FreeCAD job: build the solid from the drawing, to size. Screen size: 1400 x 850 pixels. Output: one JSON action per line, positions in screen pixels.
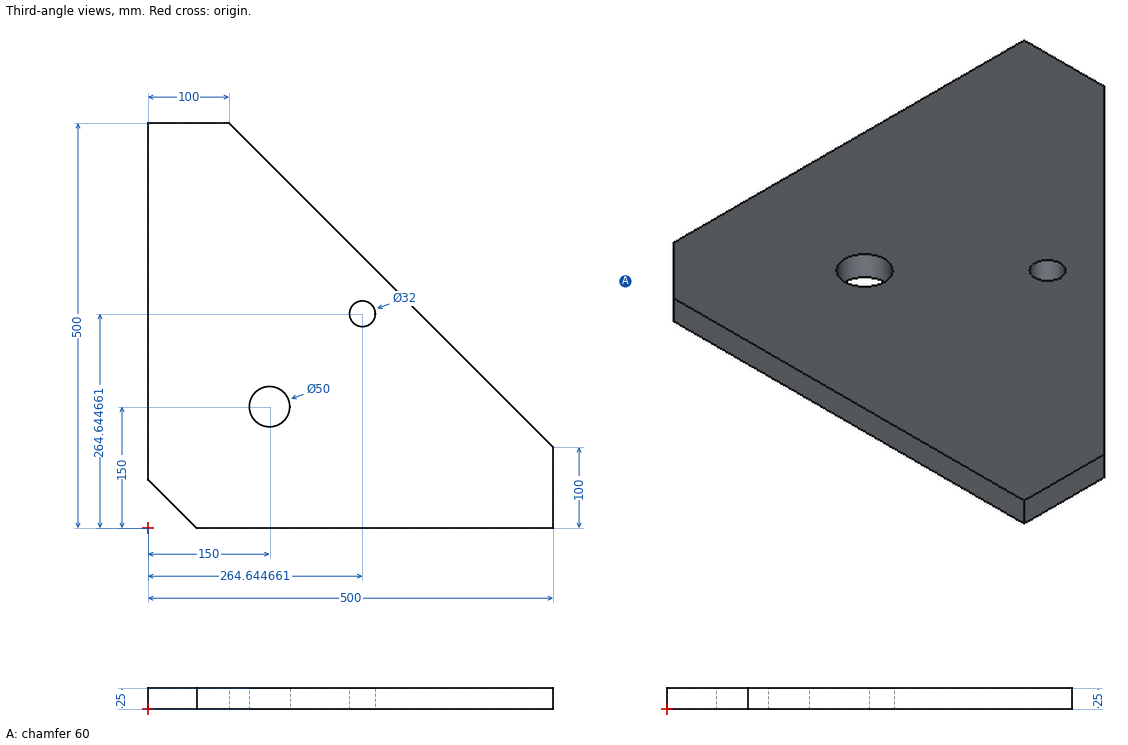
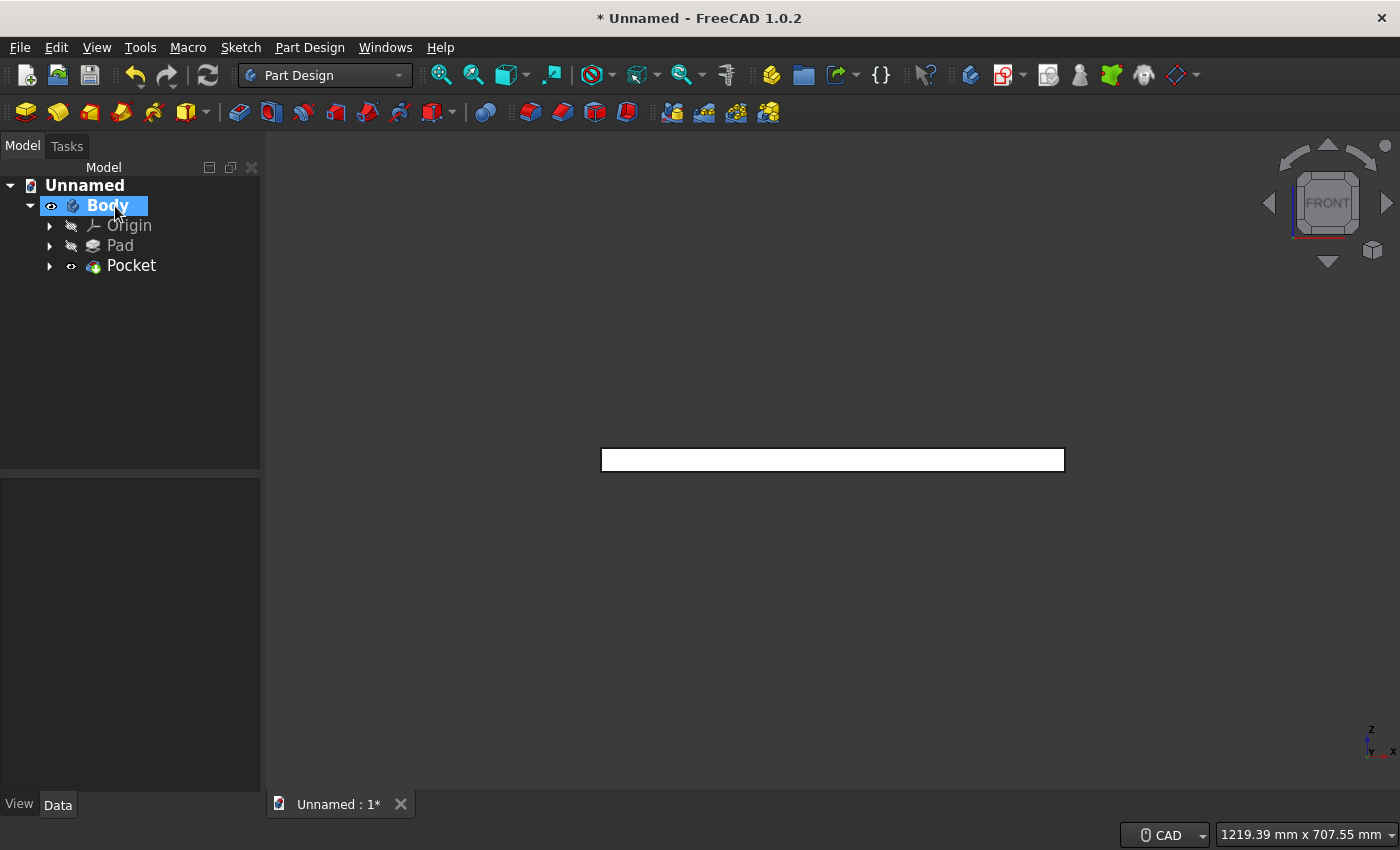
{"action": "left_click", "coordinate": [442, 76]}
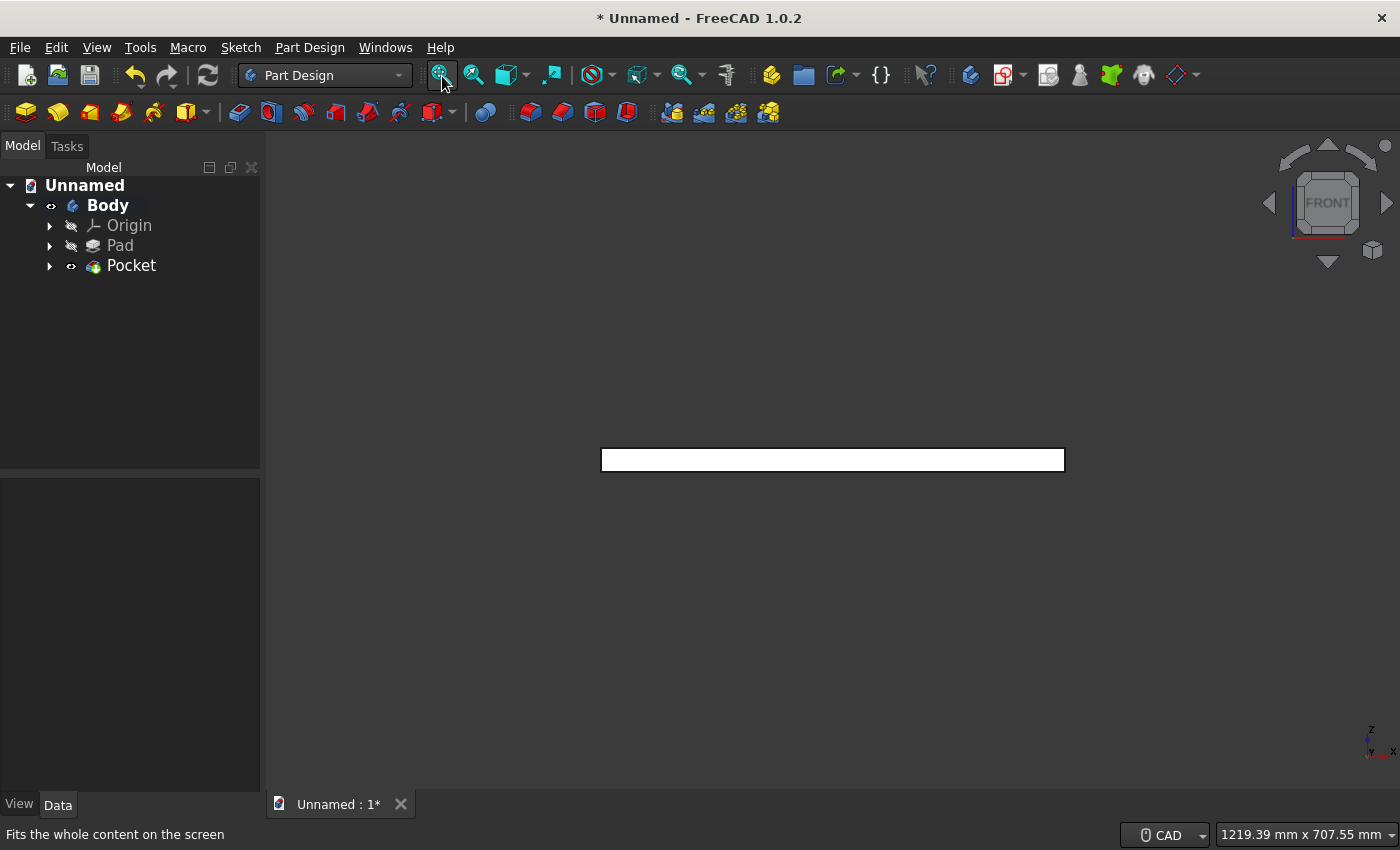
{"action": "left_click", "coordinate": [601, 459]}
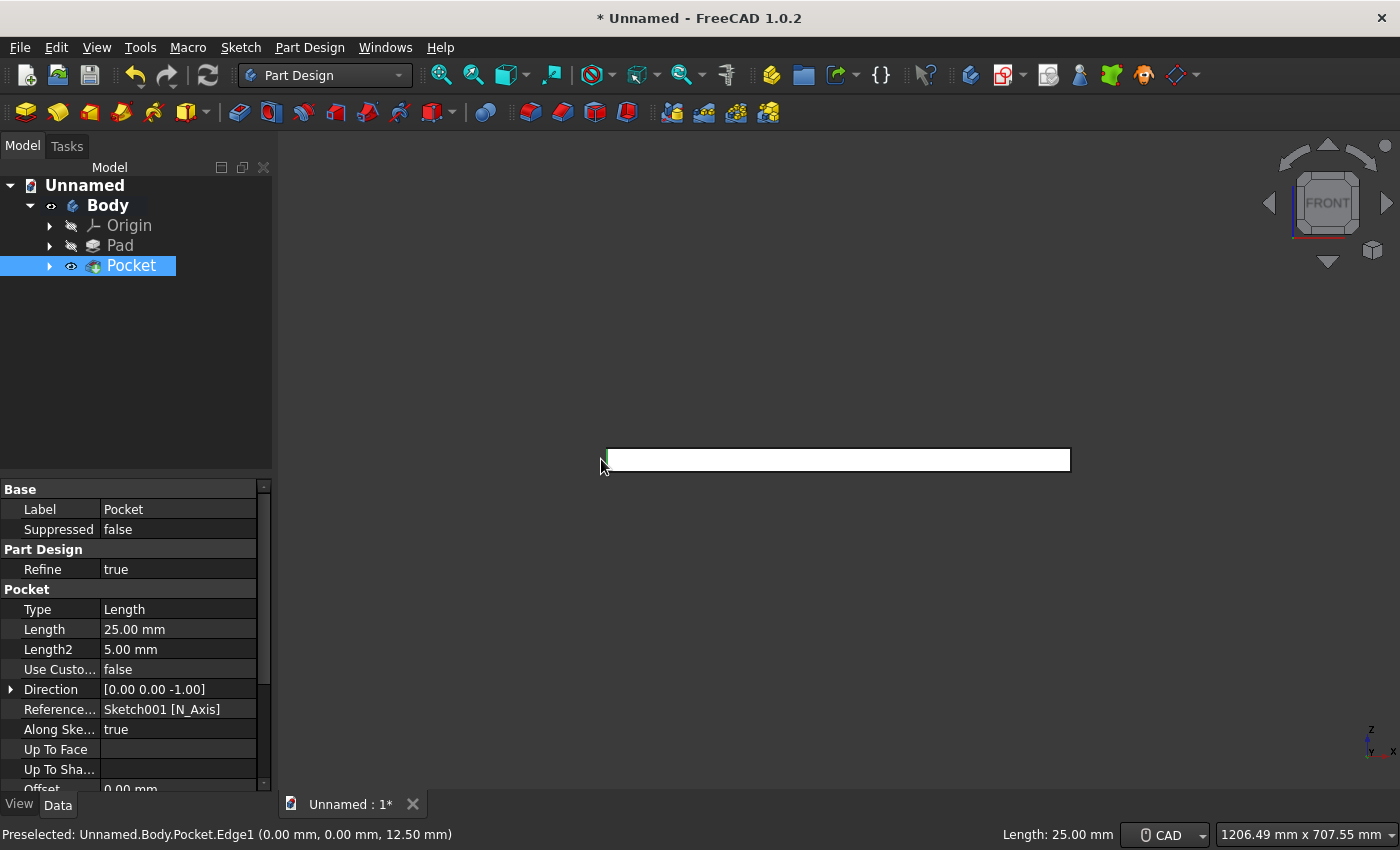
{"action": "left_click", "coordinate": [564, 112]}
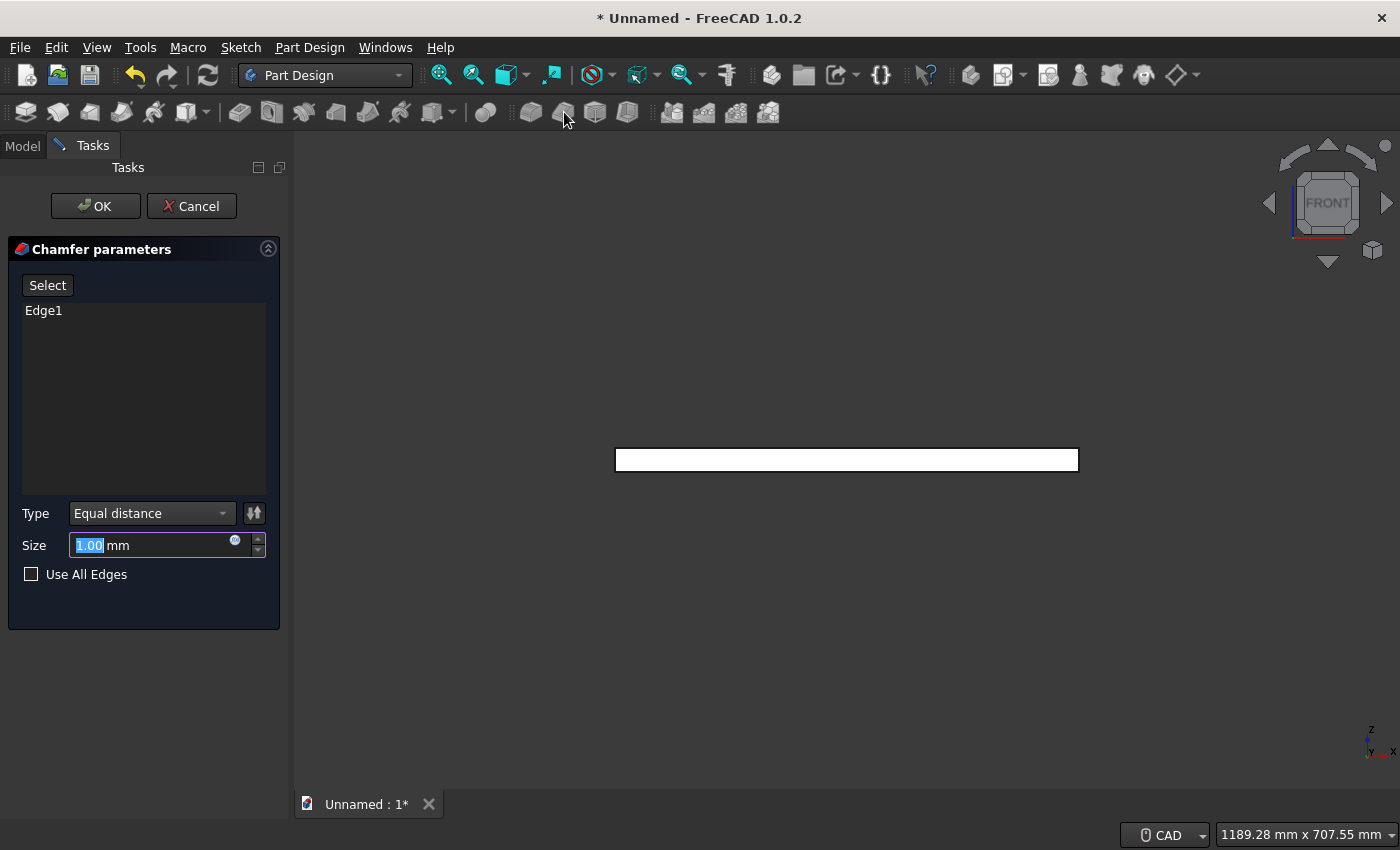
{"action": "type", "text": "60"}
{"action": "key", "text": "Tab"}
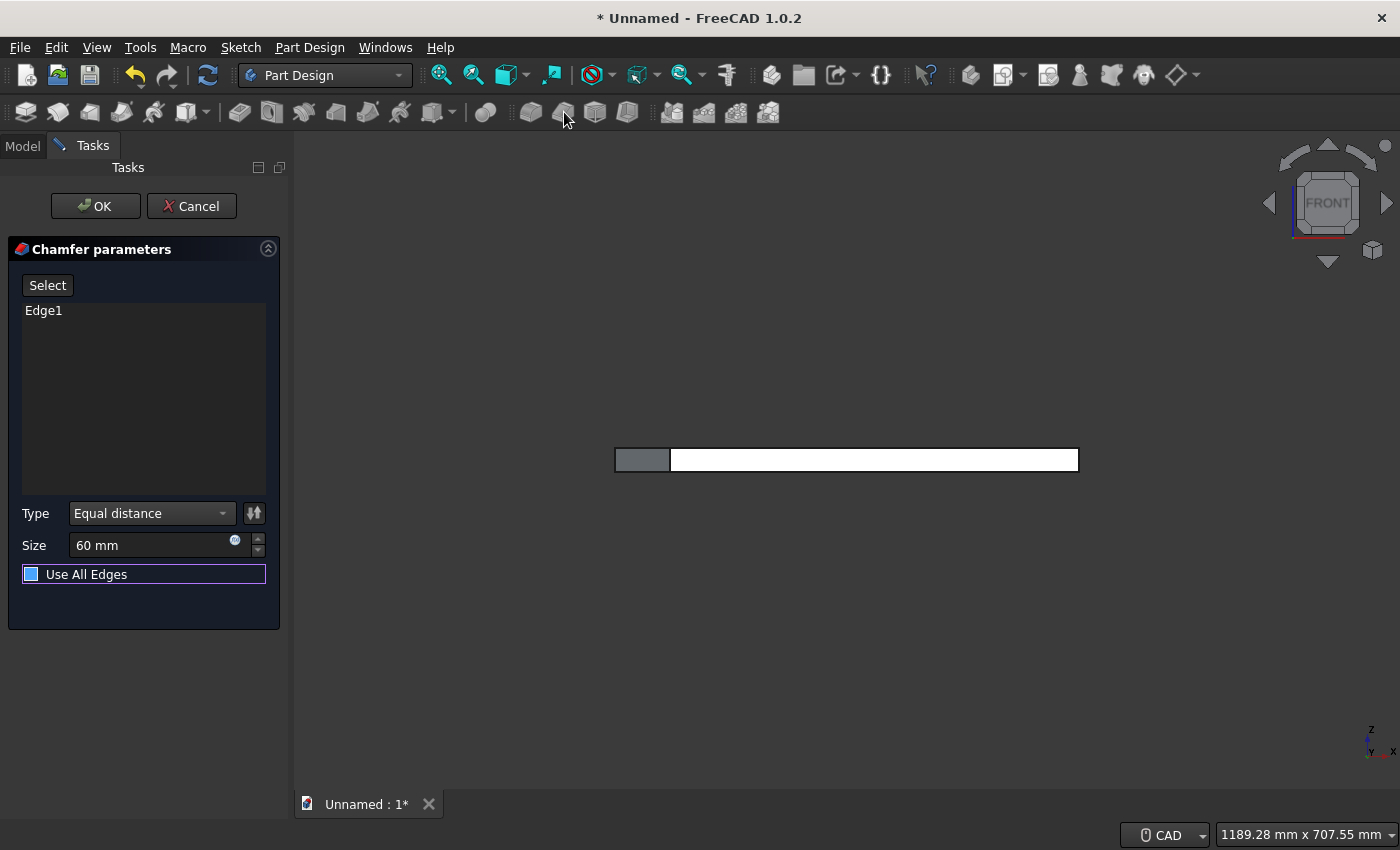
{"action": "left_click", "coordinate": [96, 206]}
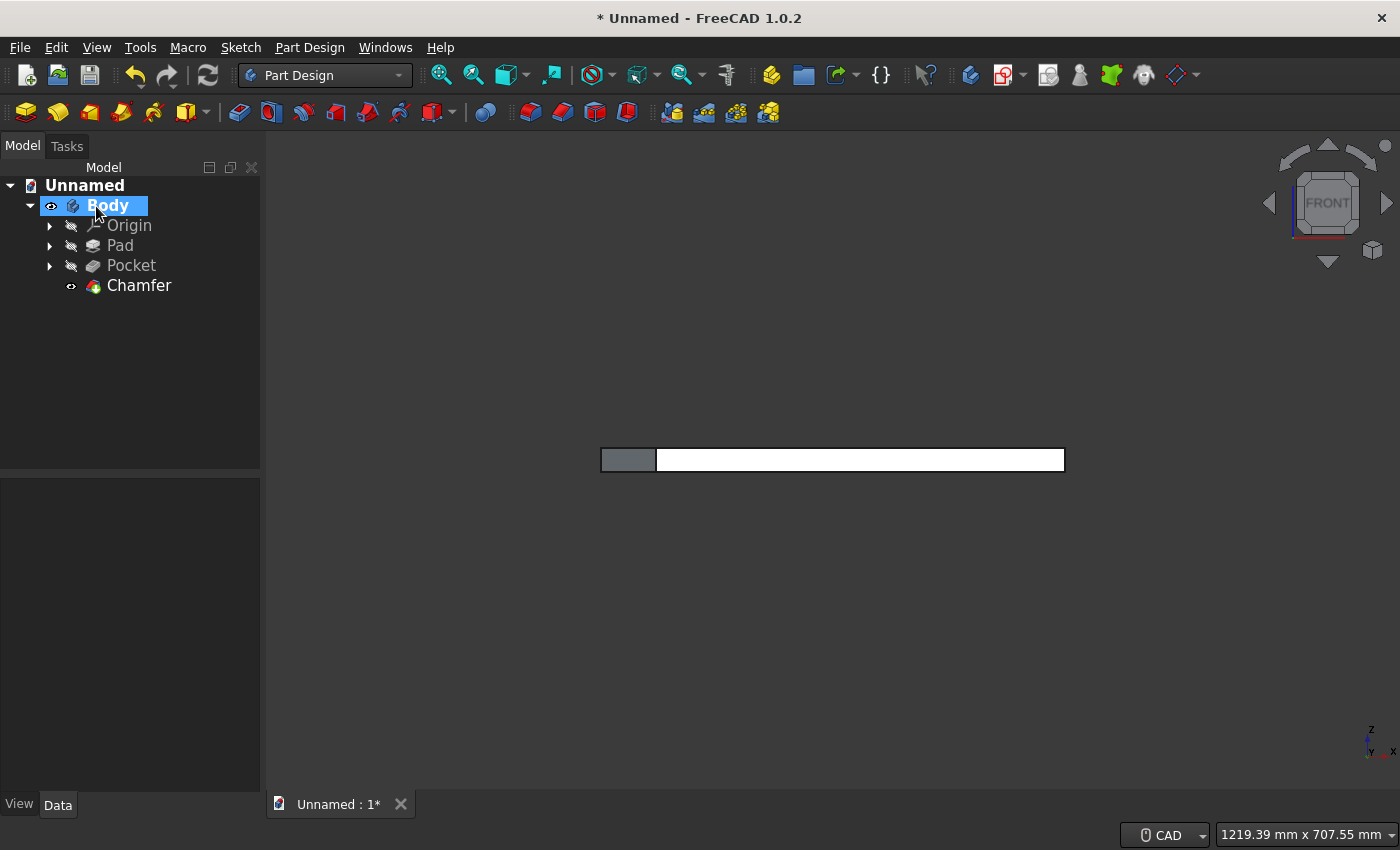
{"action": "left_click", "coordinate": [442, 76]}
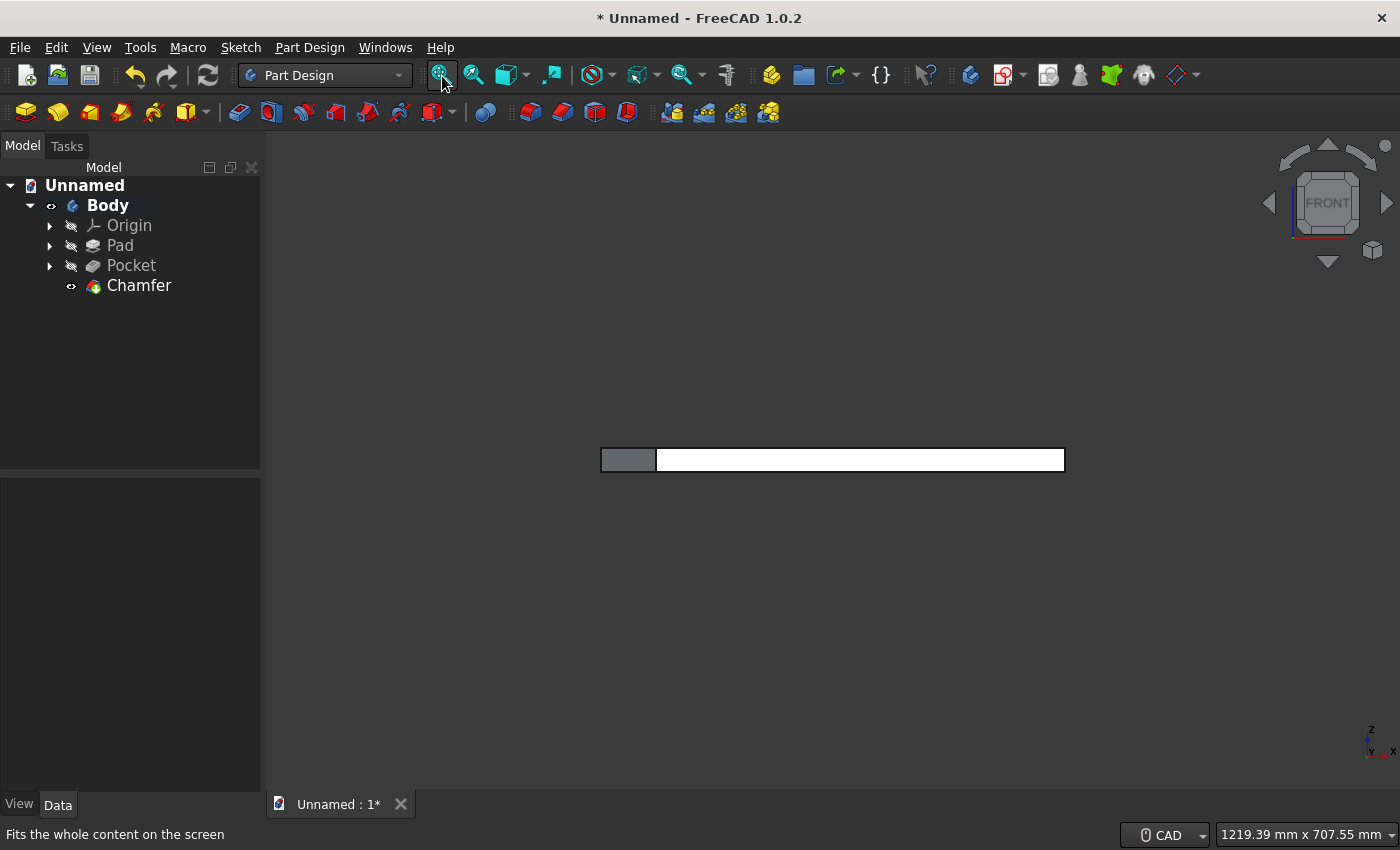
{"action": "key", "text": "0"}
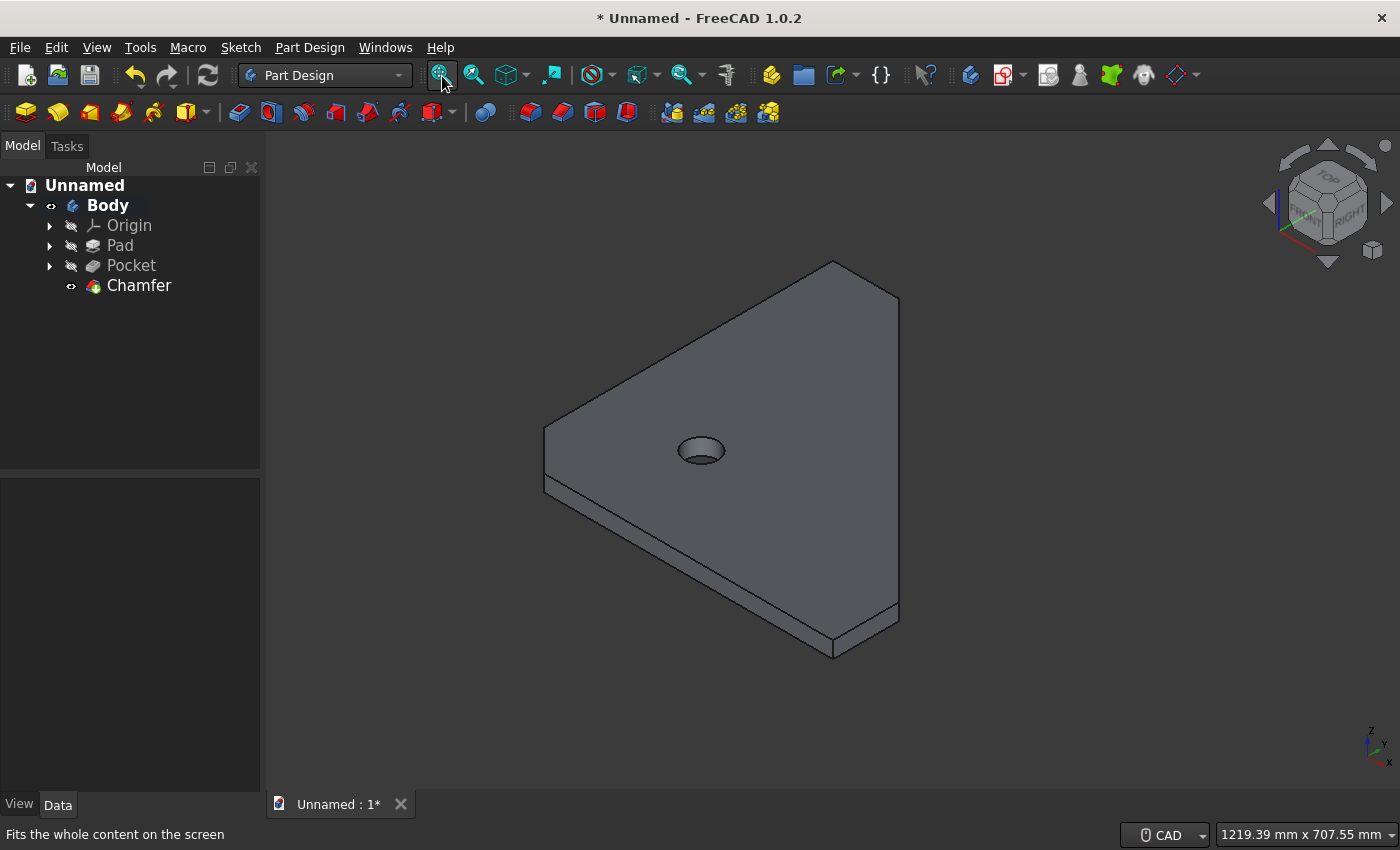
{"action": "left_click", "coordinate": [786, 531]}